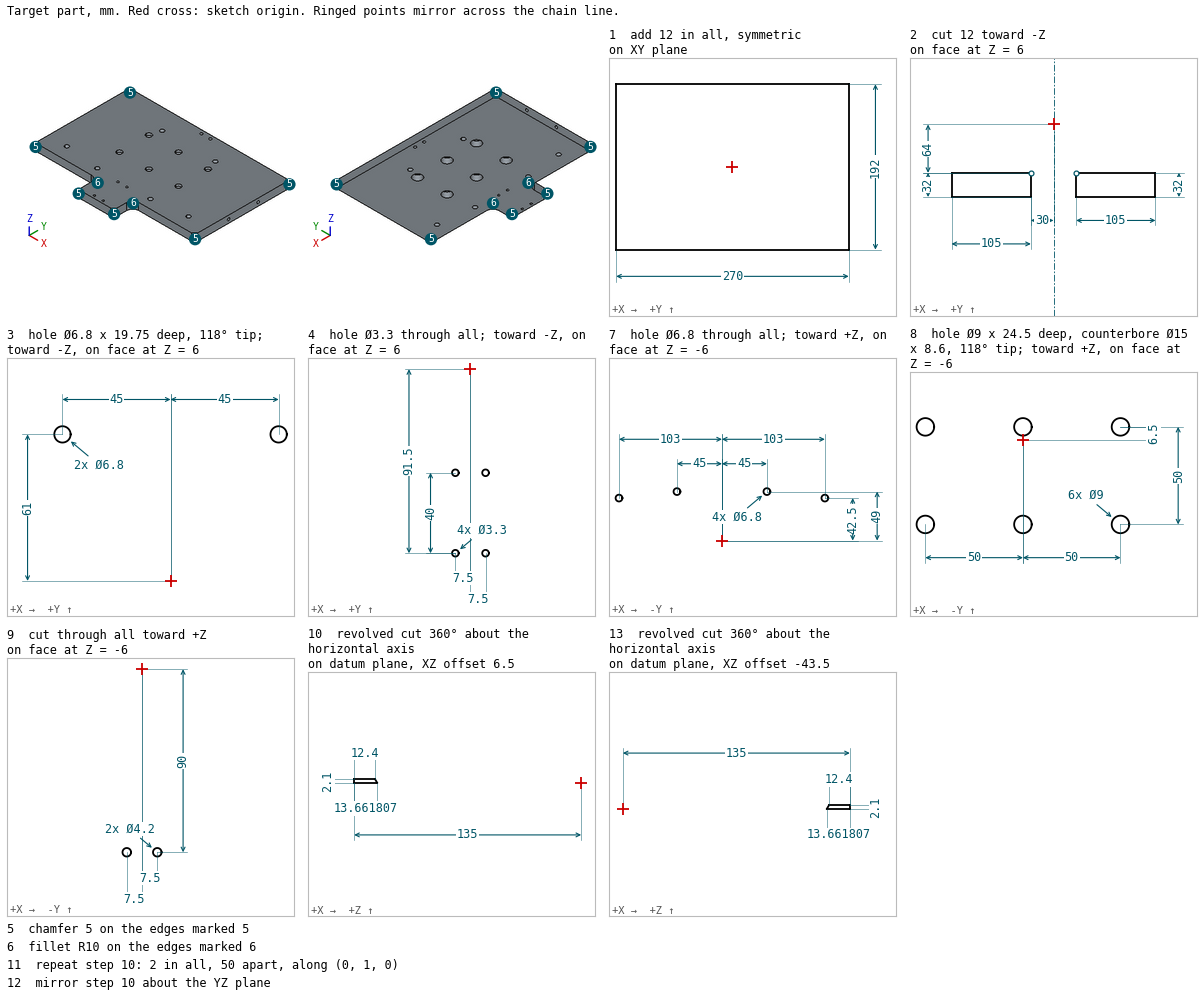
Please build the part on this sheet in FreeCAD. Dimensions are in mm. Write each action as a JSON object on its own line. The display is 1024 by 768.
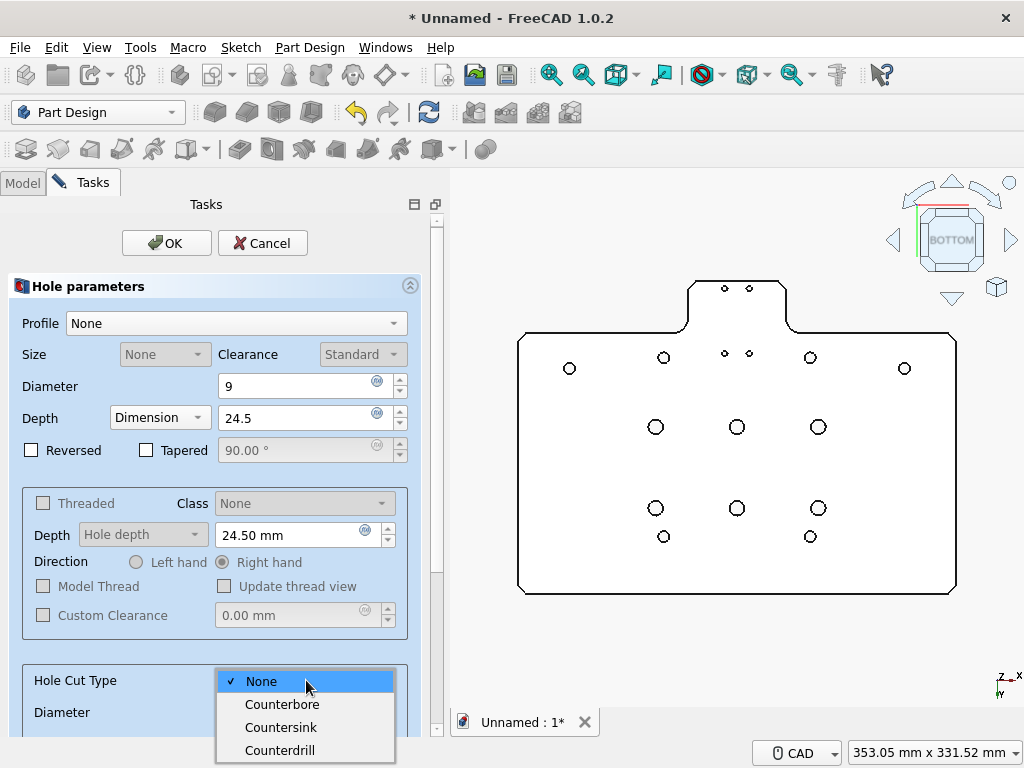
{"action": "left_click", "coordinate": [304, 704]}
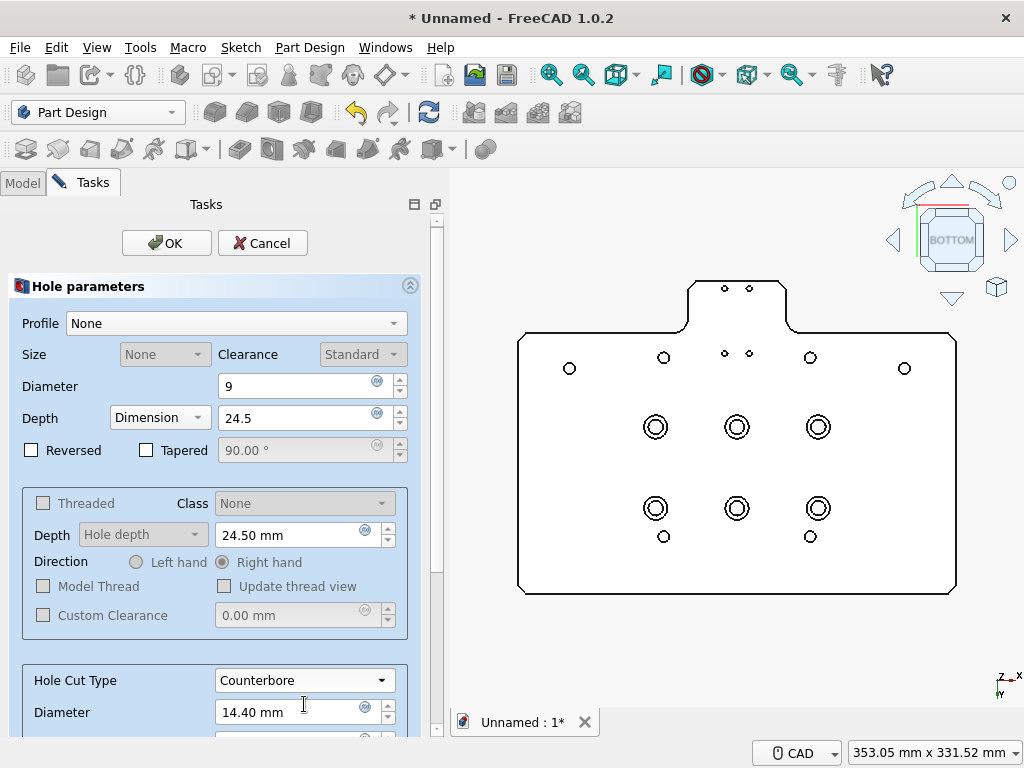
{"action": "triple_click", "coordinate": [298, 712]}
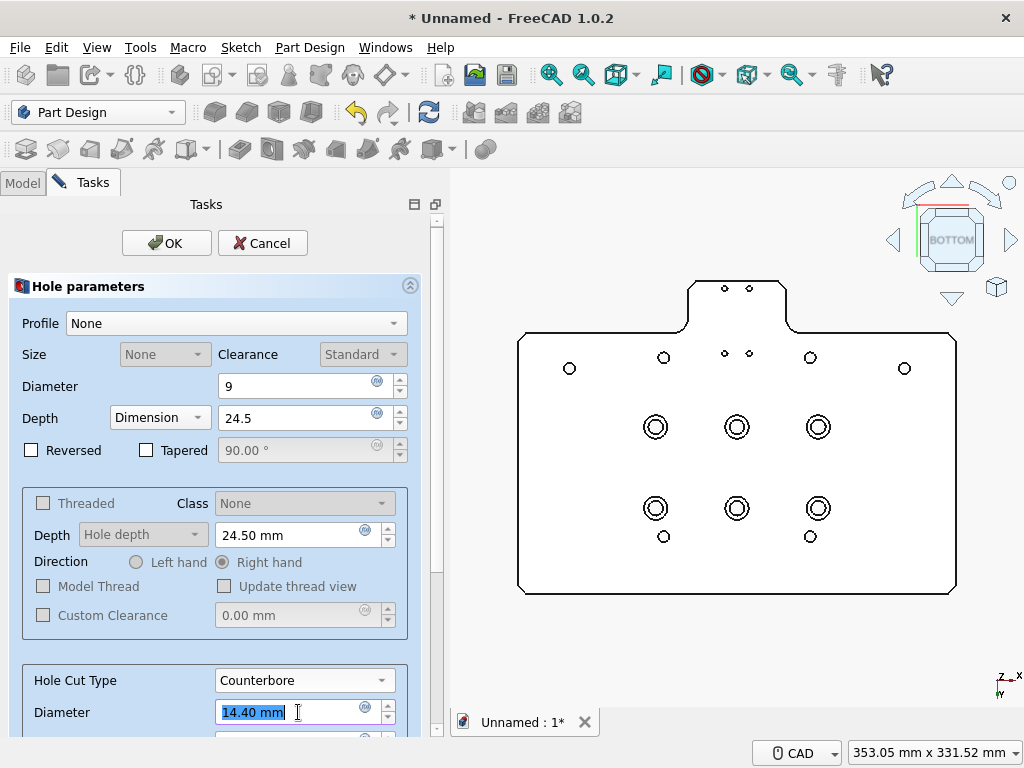
{"action": "type", "text": "15"}
{"action": "key", "text": "Tab"}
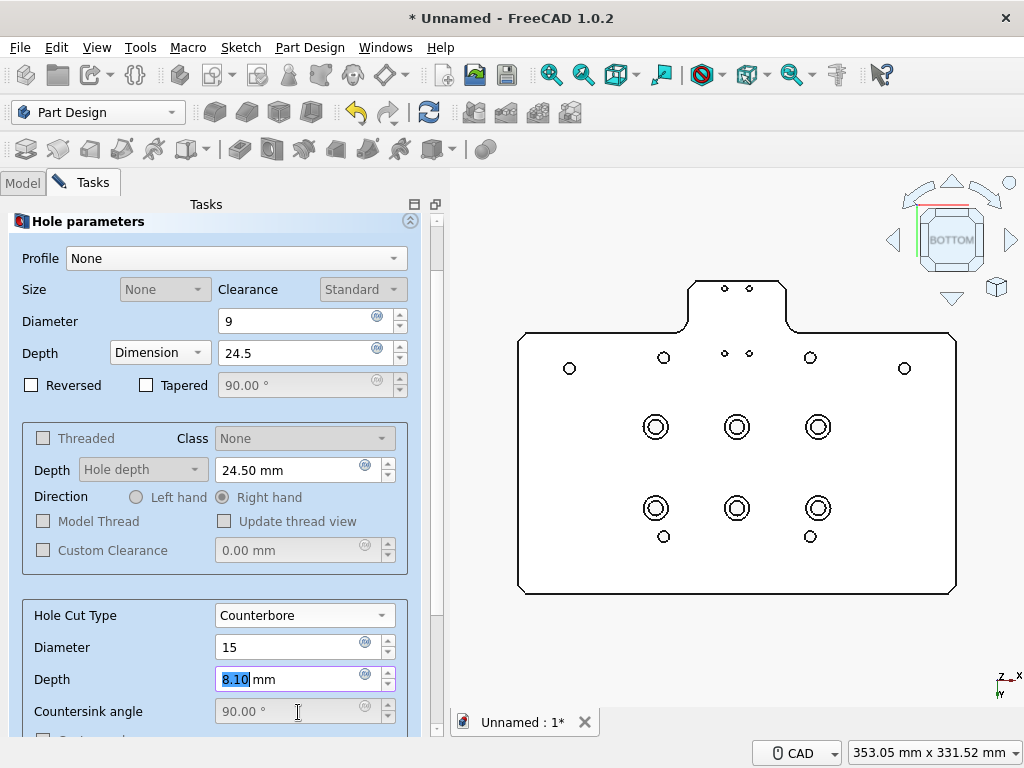
{"action": "type", "text": "8.6"}
{"action": "key", "text": "Tab"}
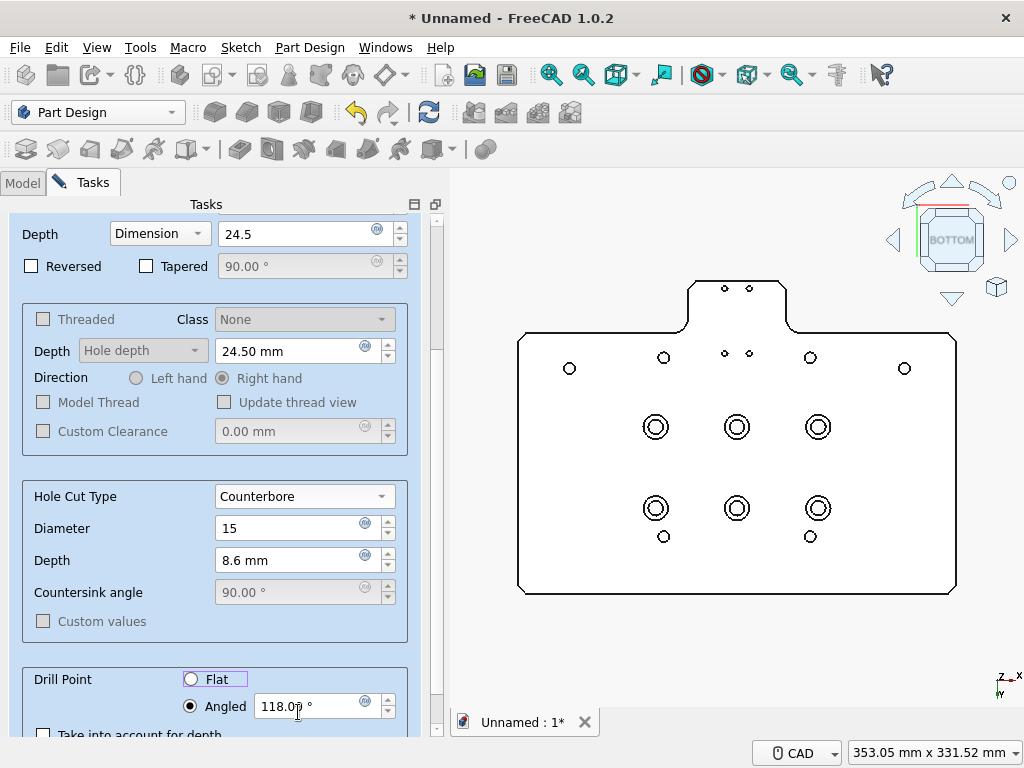
{"action": "scroll", "coordinate": [437, 475], "scroll_direction": "up", "scroll_amount": 4}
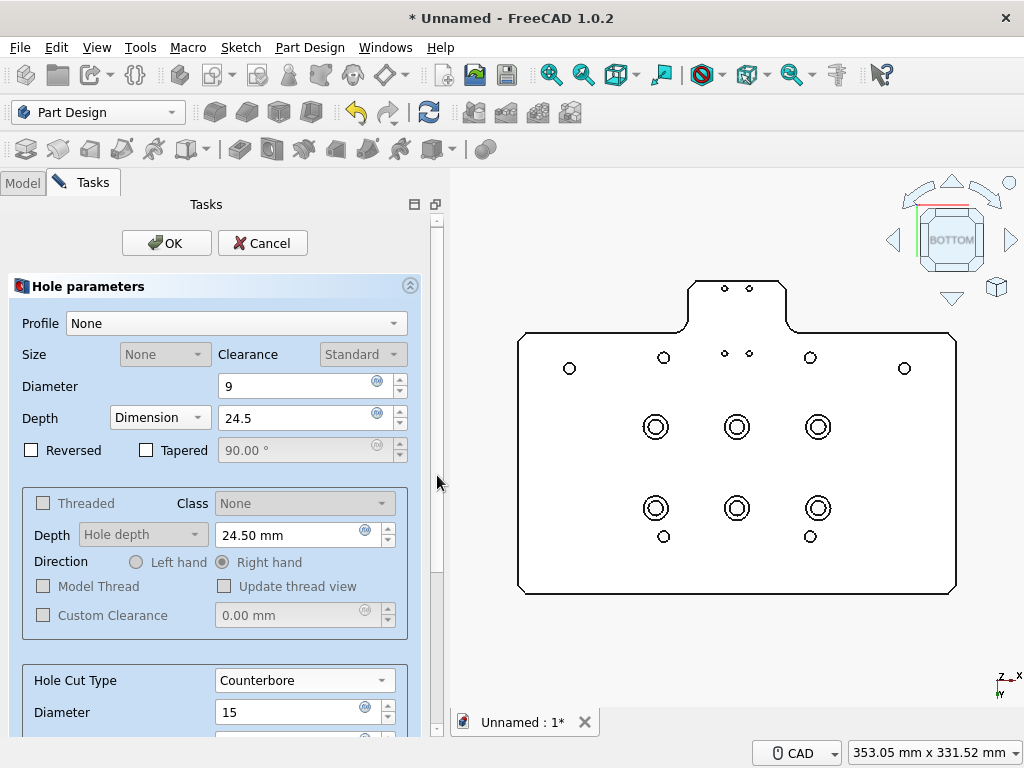
{"action": "left_click", "coordinate": [167, 243]}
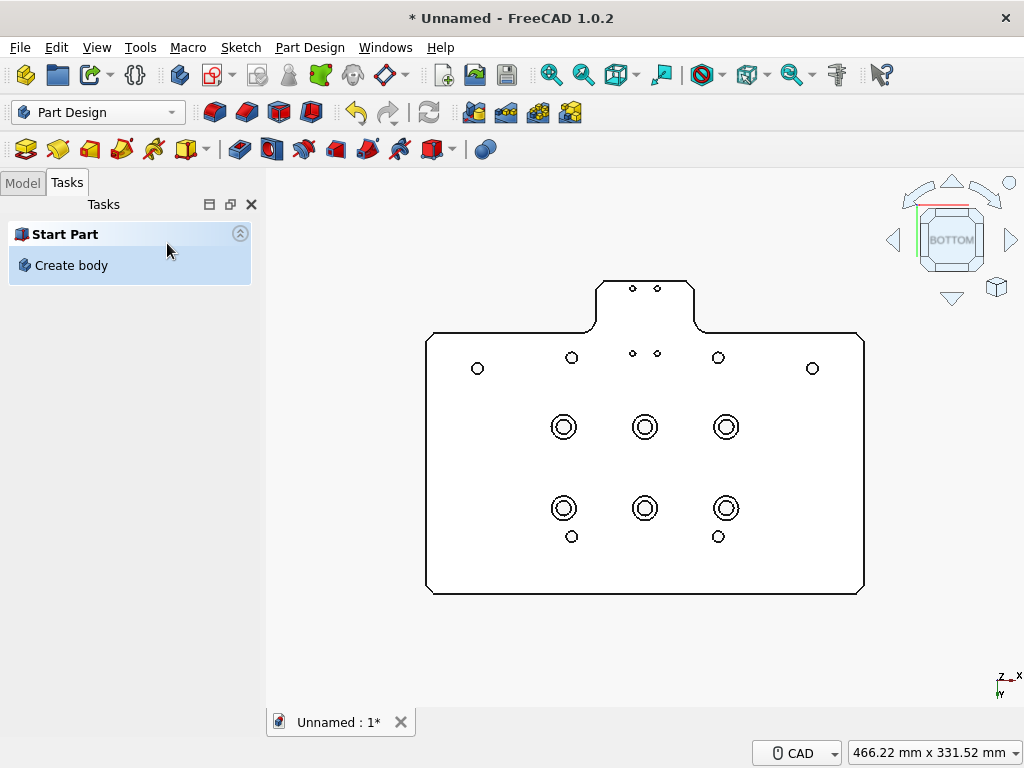
{"action": "left_click", "coordinate": [770, 392]}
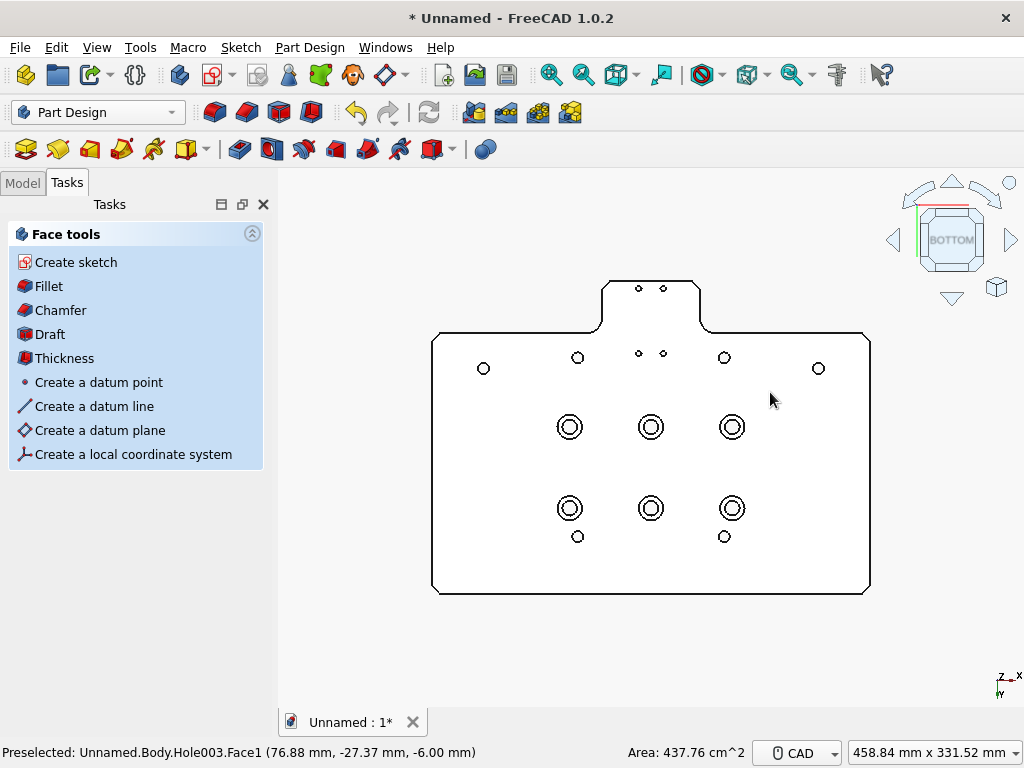
{"action": "left_click", "coordinate": [212, 76]}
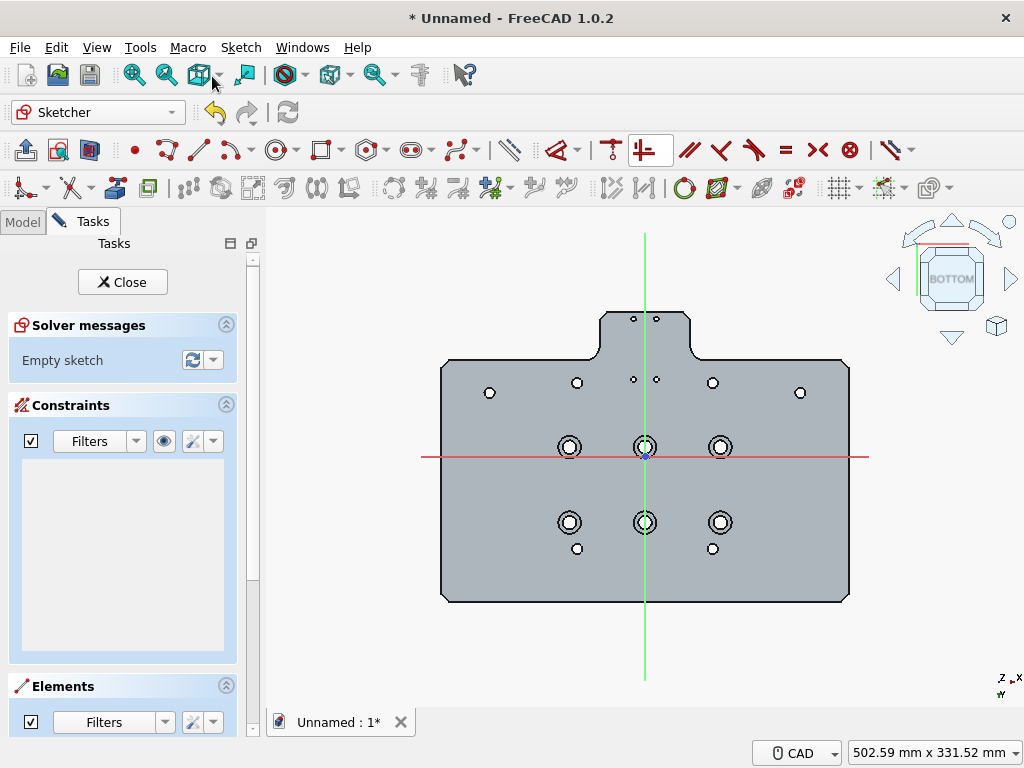
{"action": "scroll", "coordinate": [650, 604], "scroll_direction": "up", "scroll_amount": 13}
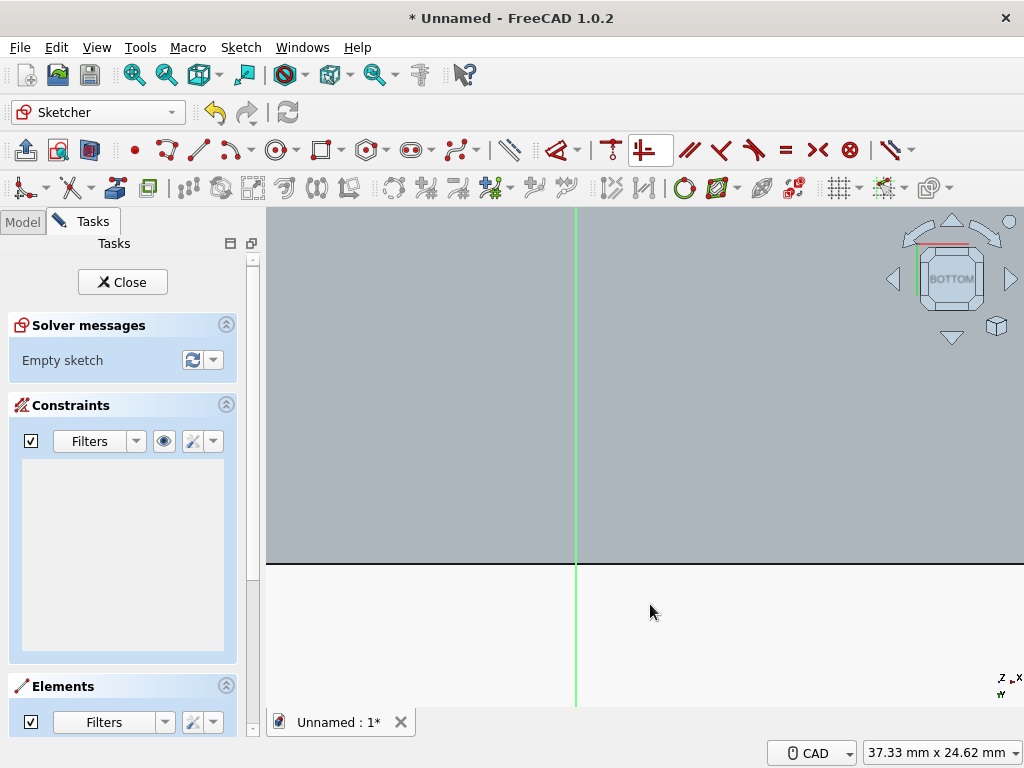
{"action": "key", "text": "g c"}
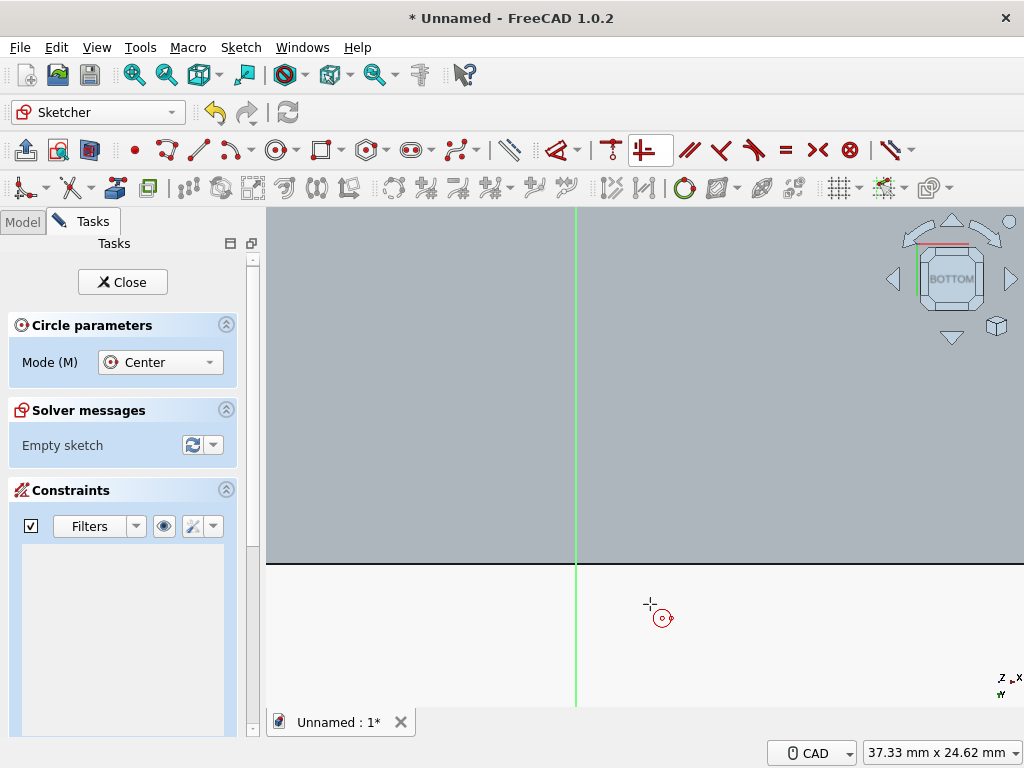
{"action": "left_click", "coordinate": [729, 442]}
{"action": "mouse_move", "coordinate": [759, 412]}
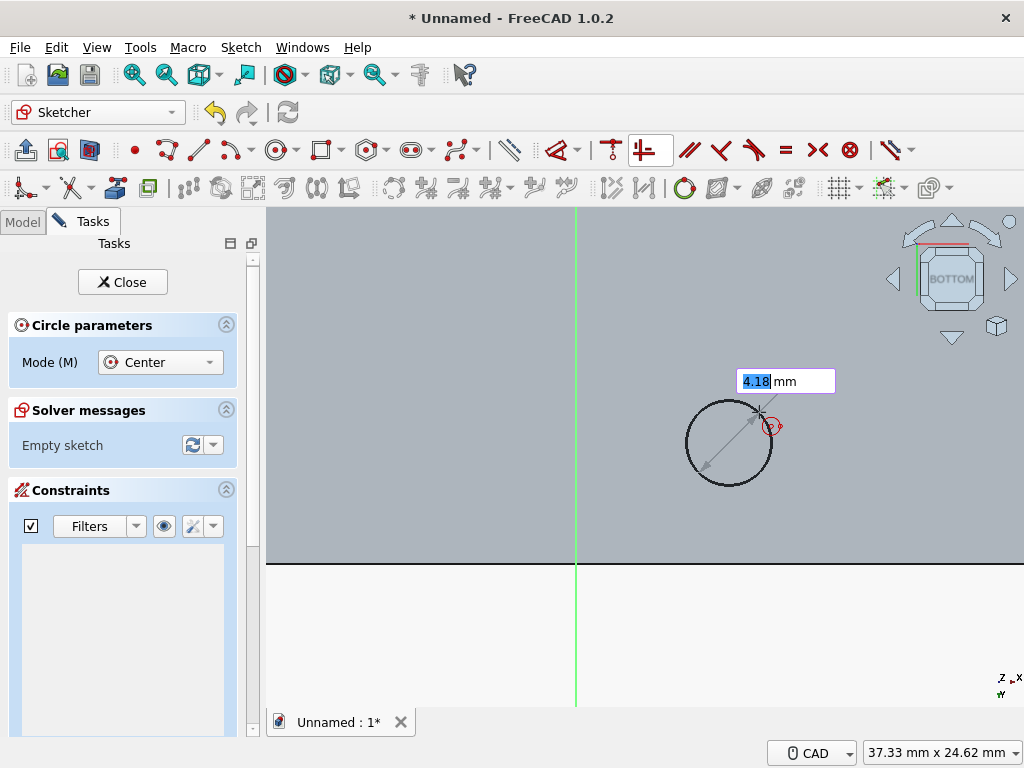
{"action": "type", "text": "4.2"}
{"action": "key", "text": "Return"}